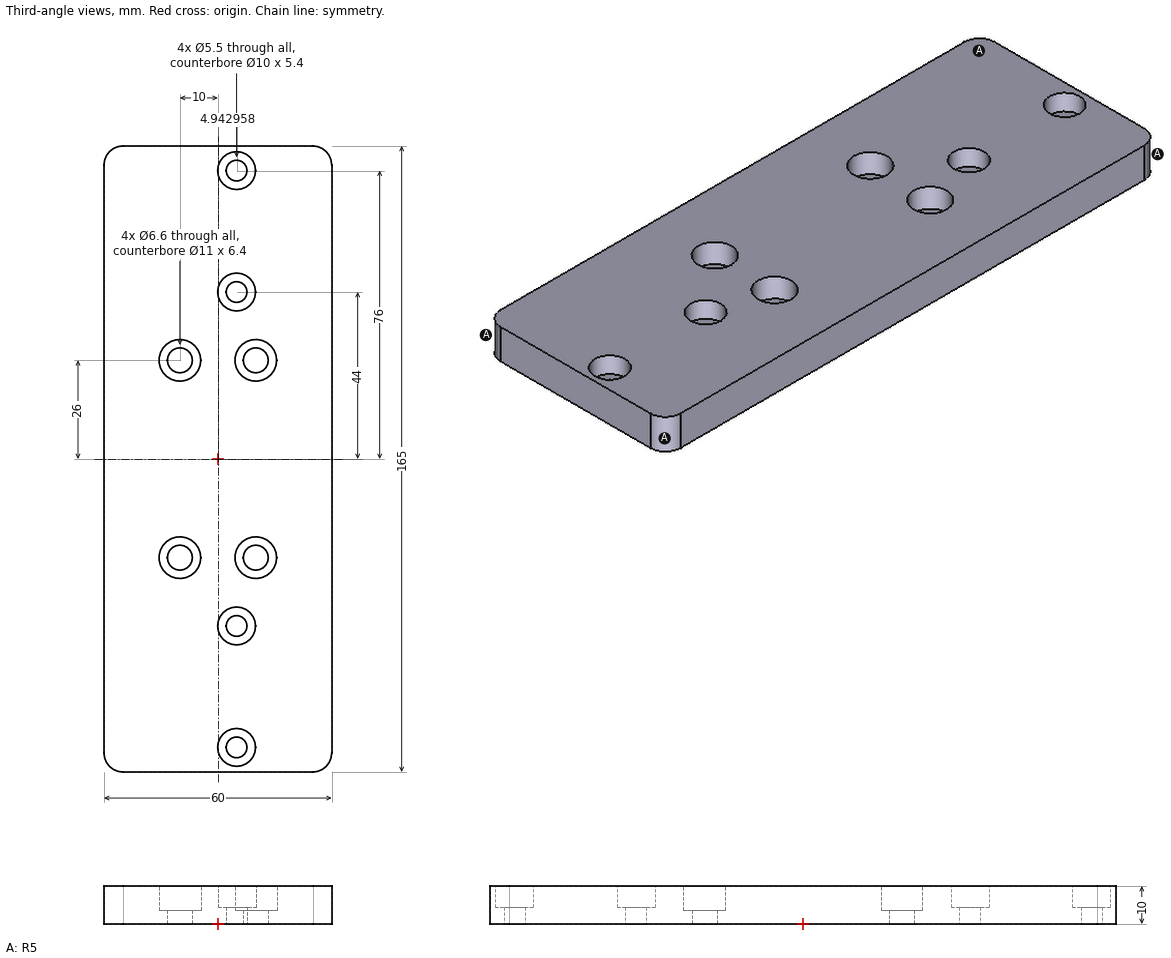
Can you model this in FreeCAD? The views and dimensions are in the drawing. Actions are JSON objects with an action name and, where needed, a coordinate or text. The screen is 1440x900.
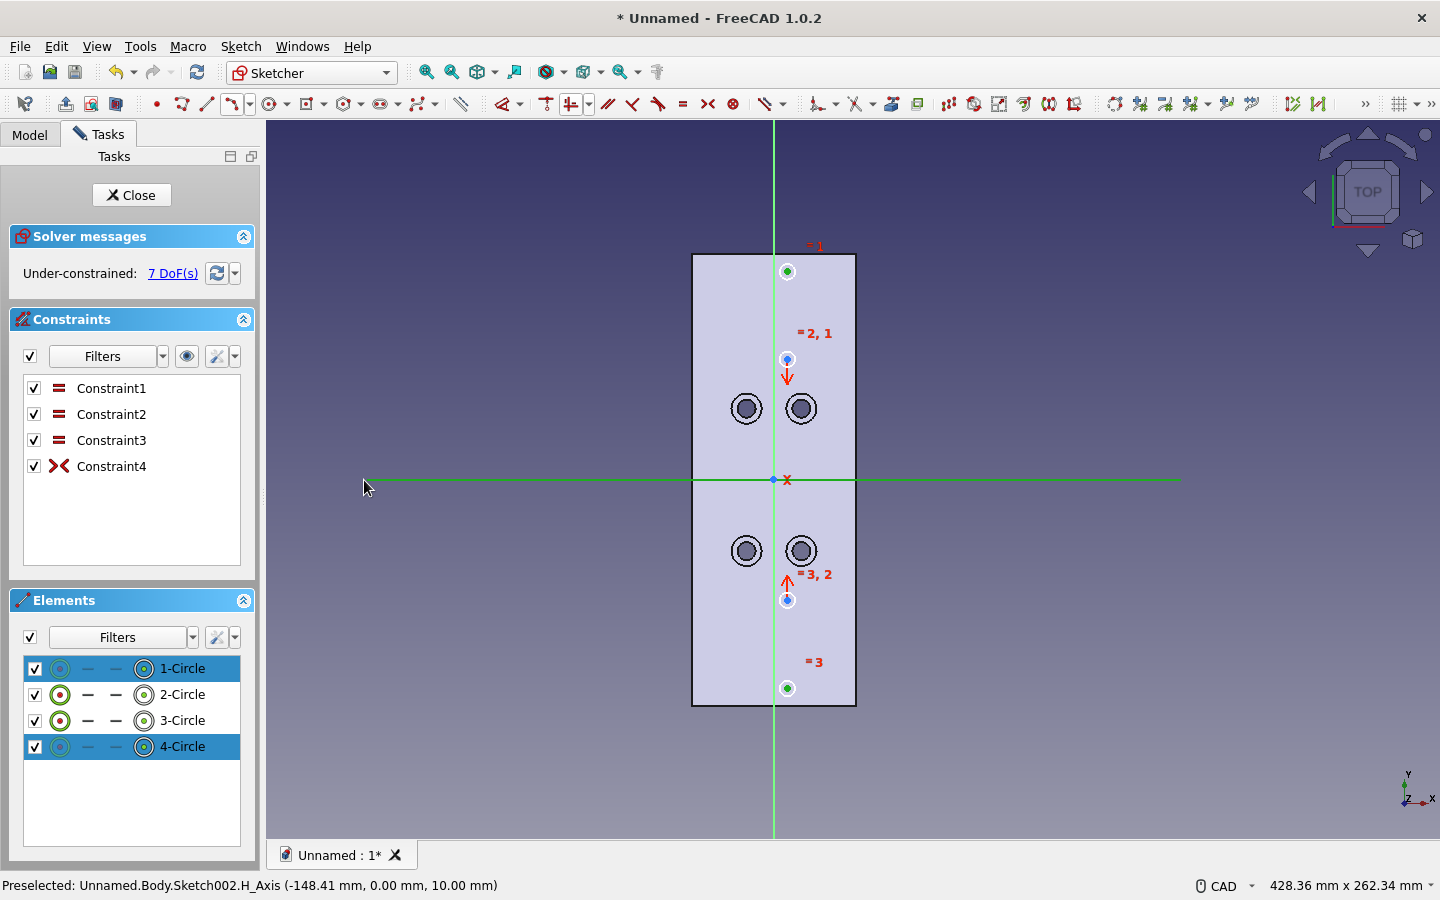
{"action": "left_click", "coordinate": [708, 104]}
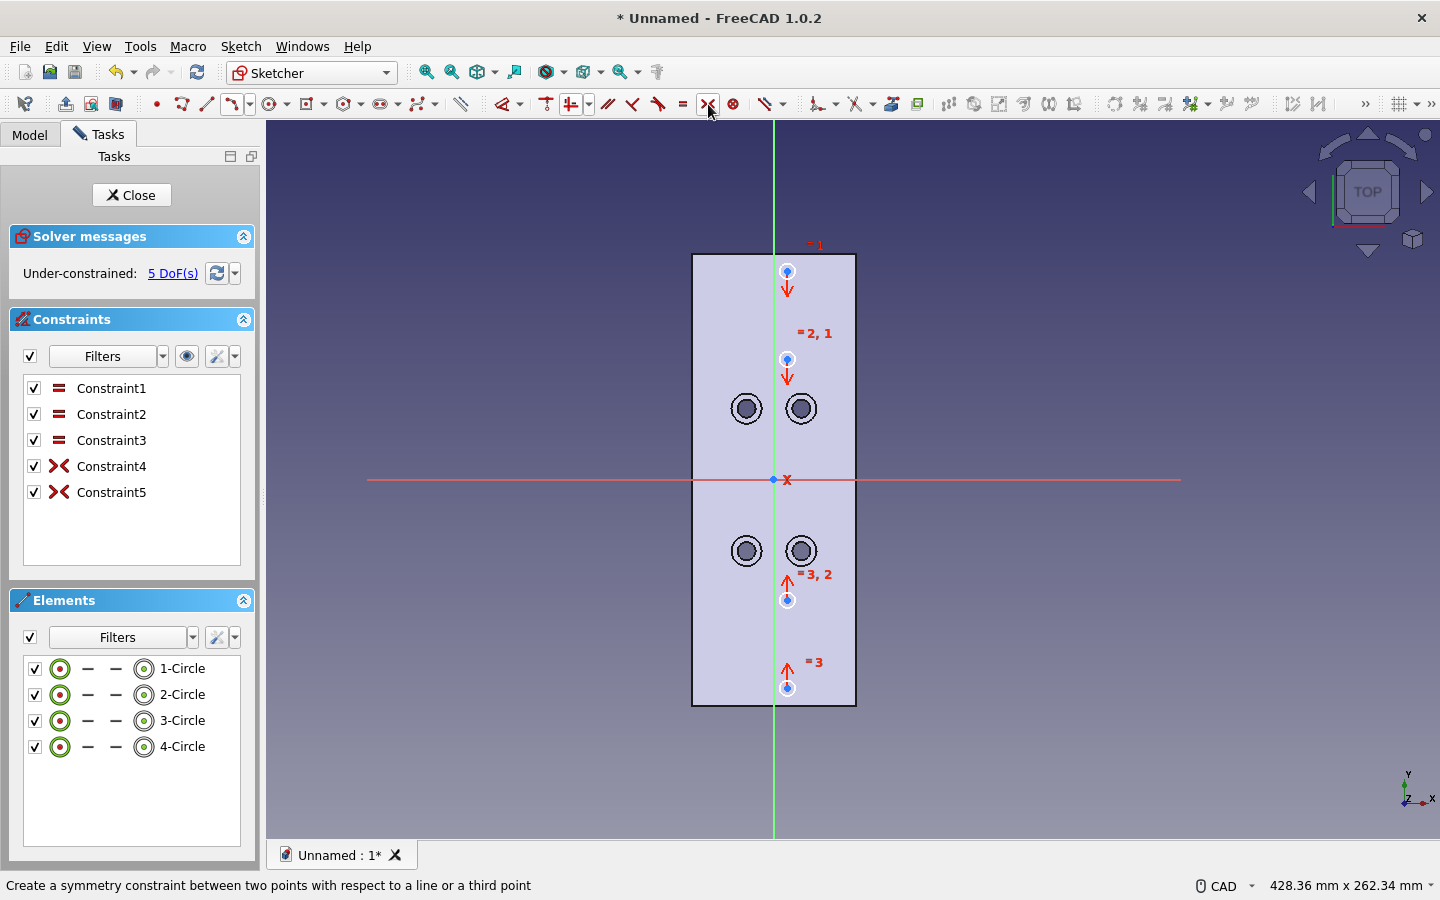
{"action": "left_click", "coordinate": [502, 104]}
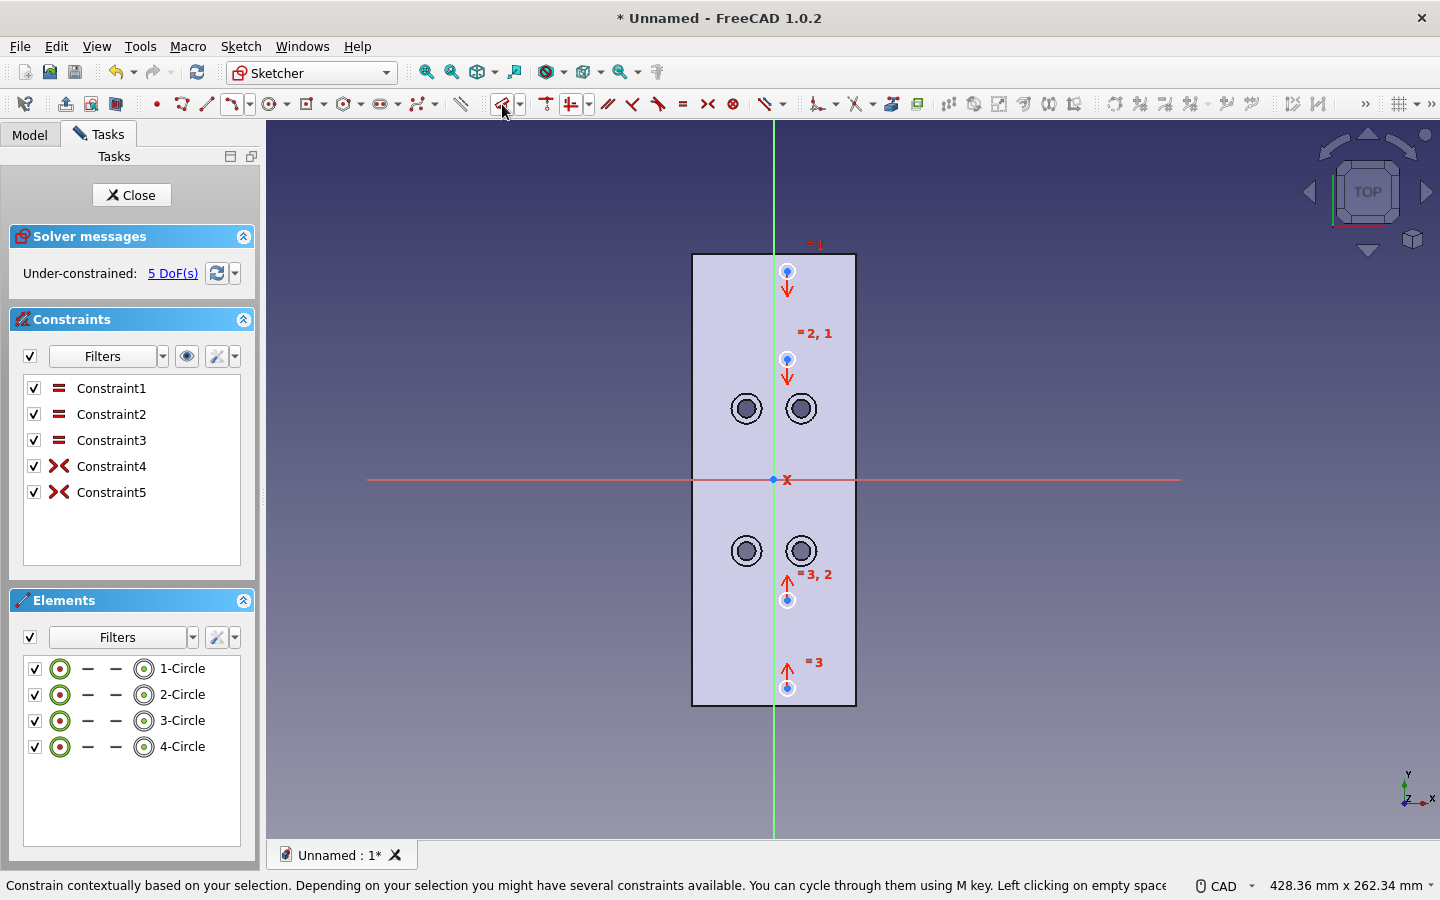
{"action": "scroll", "coordinate": [782, 266], "scroll_direction": "up", "scroll_amount": 5}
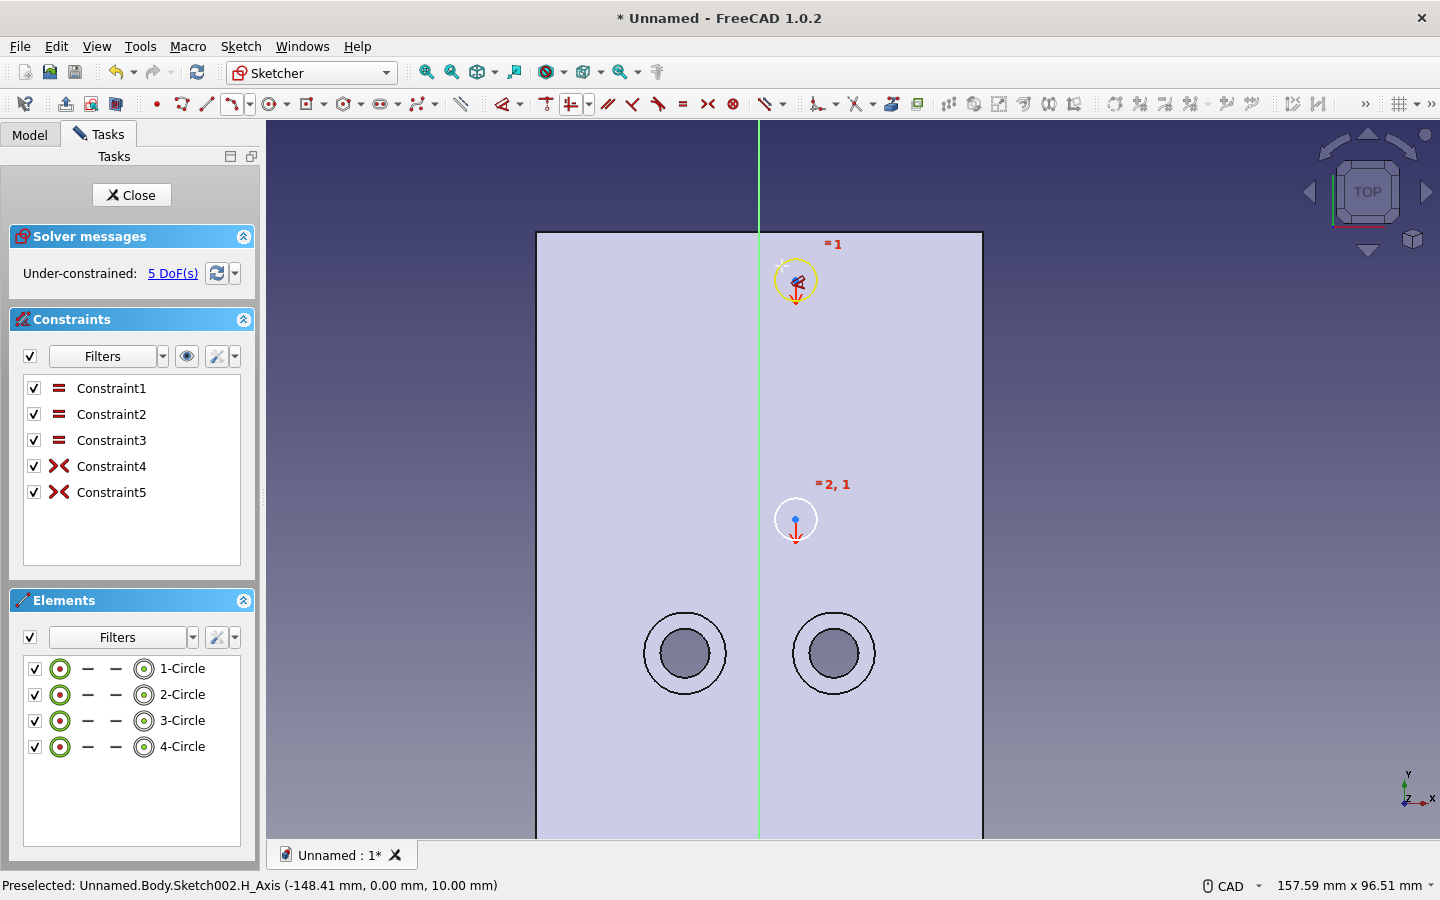
{"action": "left_click", "coordinate": [781, 265]}
{"action": "left_click", "coordinate": [781, 229]}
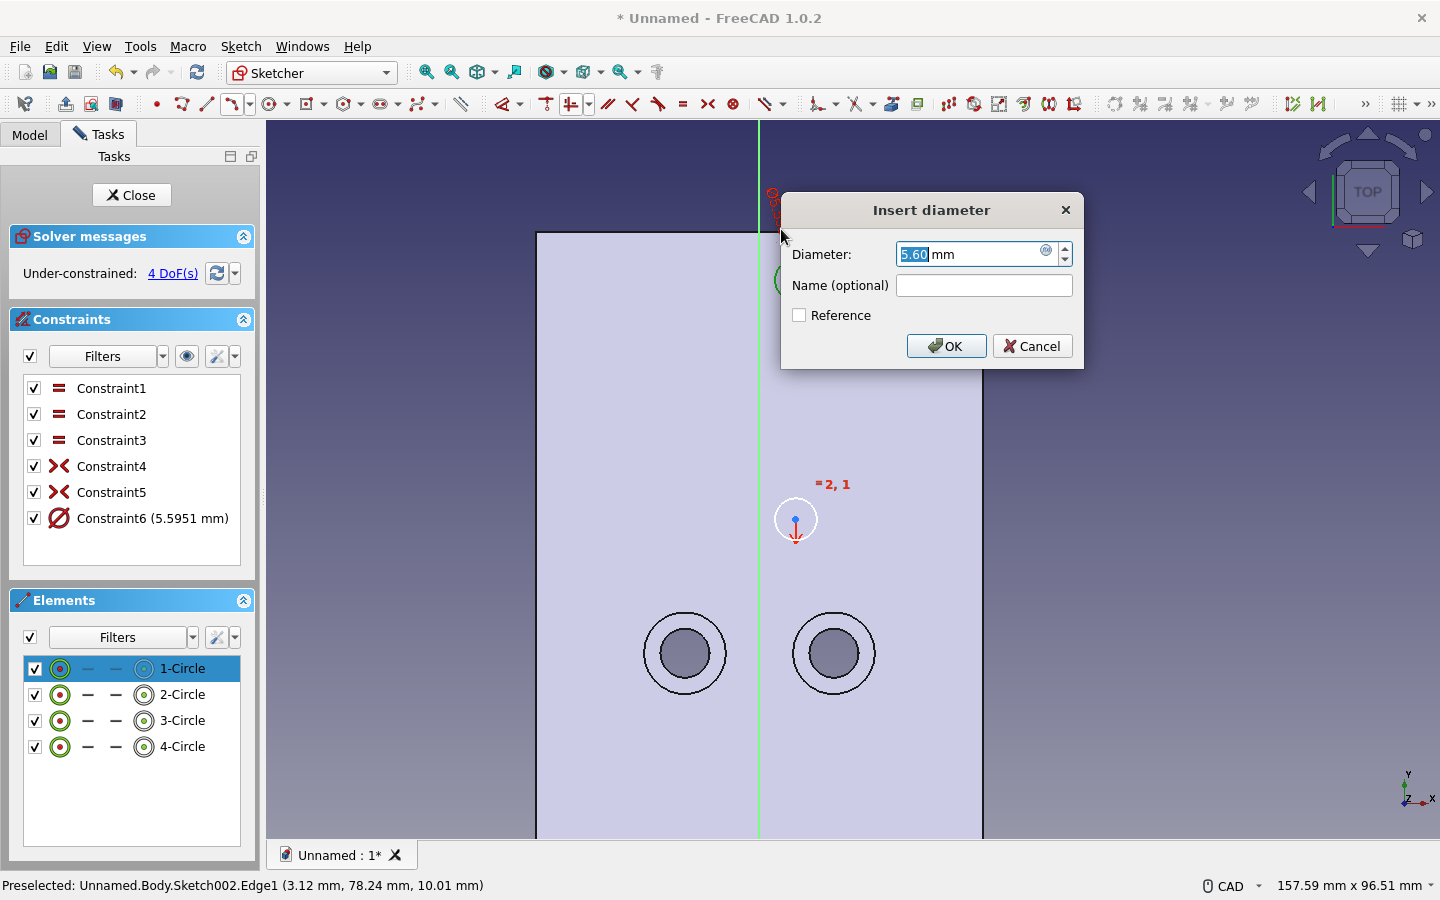
{"action": "type", "text": "5.5"}
{"action": "key", "text": "Return"}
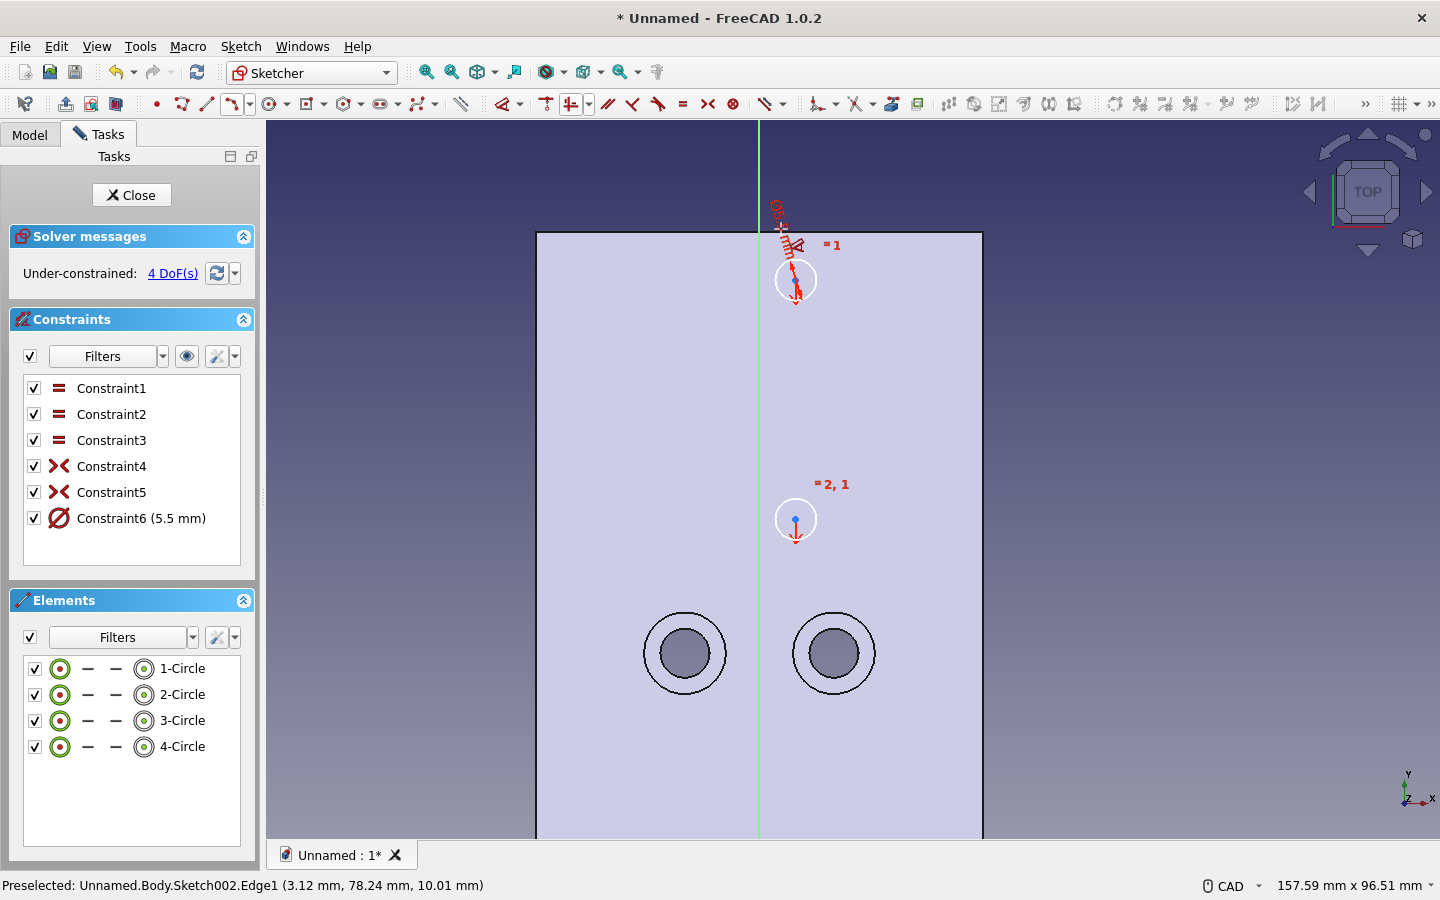
{"action": "left_click", "coordinate": [796, 280]}
{"action": "left_click", "coordinate": [725, 546]}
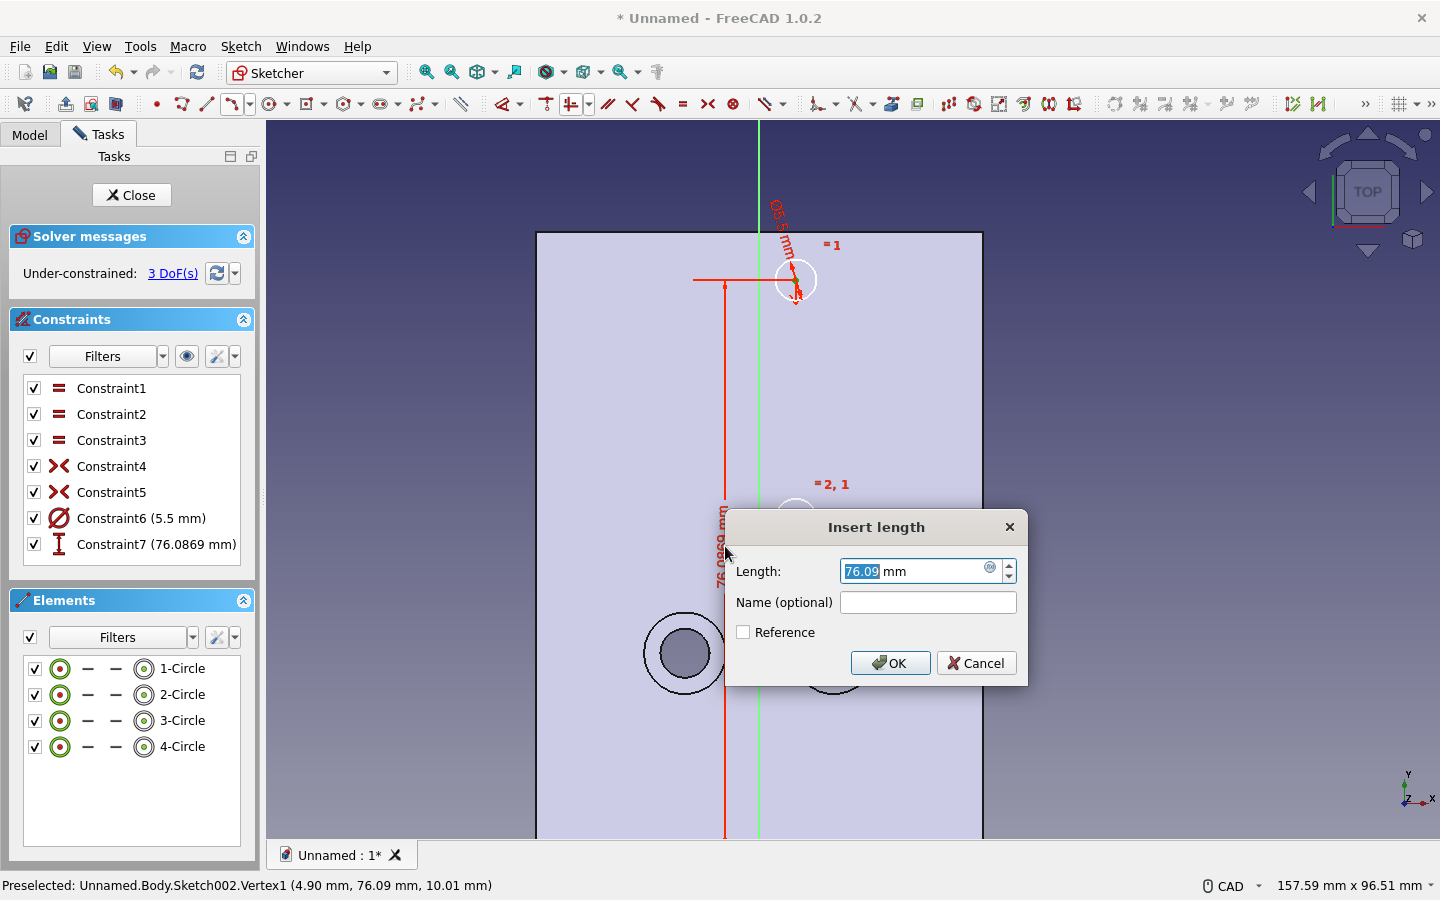
{"action": "type", "text": "76"}
{"action": "key", "text": "Return"}